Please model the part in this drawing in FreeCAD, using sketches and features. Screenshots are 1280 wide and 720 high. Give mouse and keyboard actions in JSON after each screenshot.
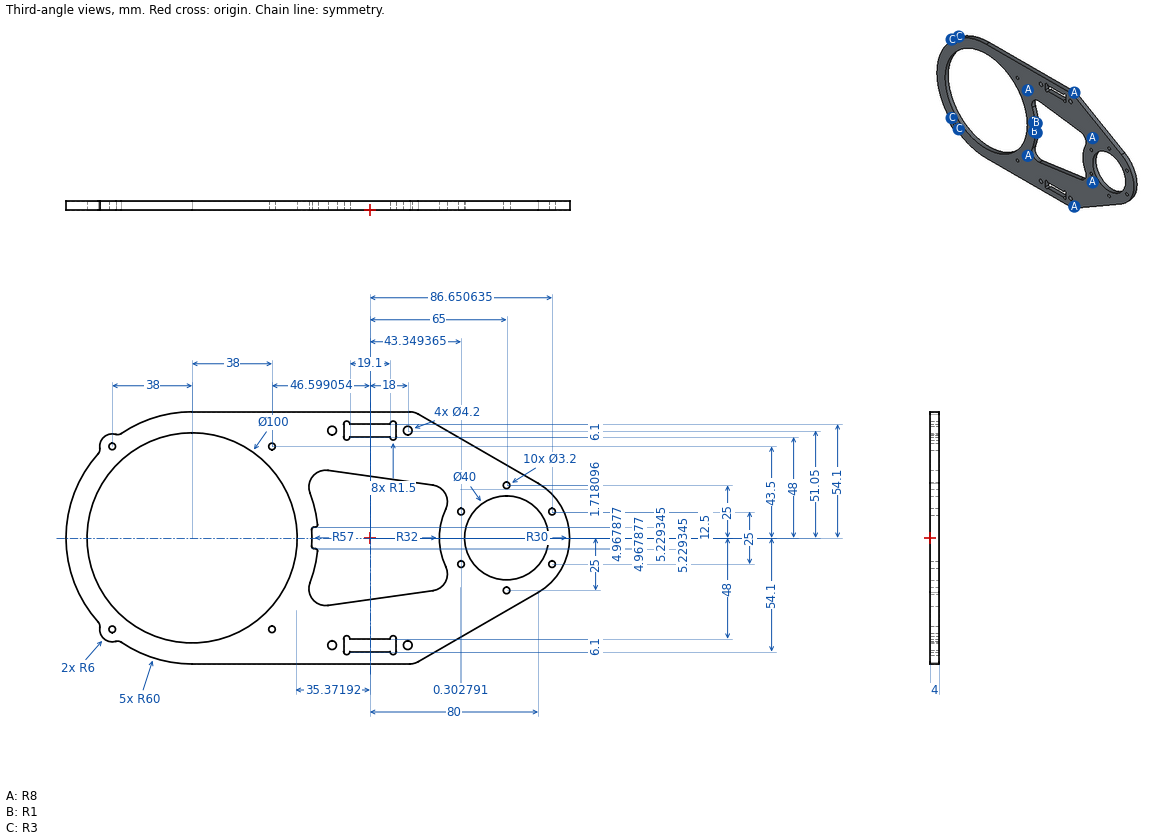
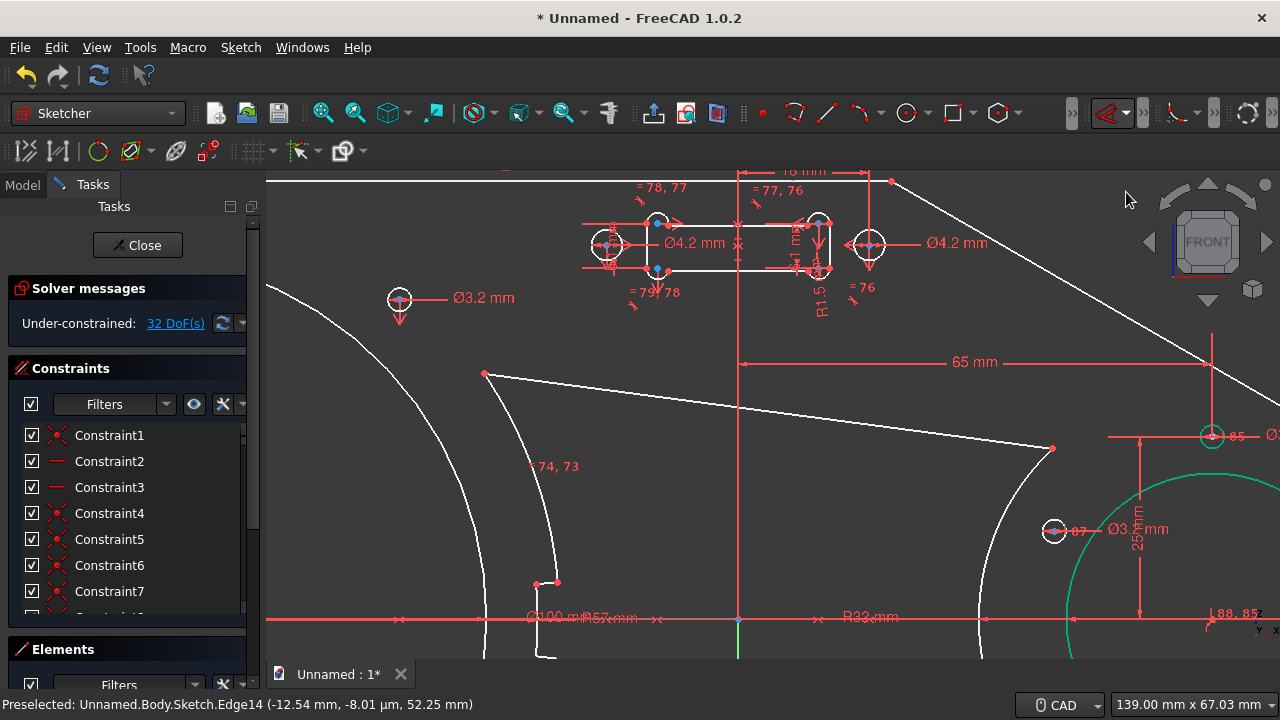
{"action": "scroll", "coordinate": [768, 326], "scroll_direction": "down", "scroll_amount": 6}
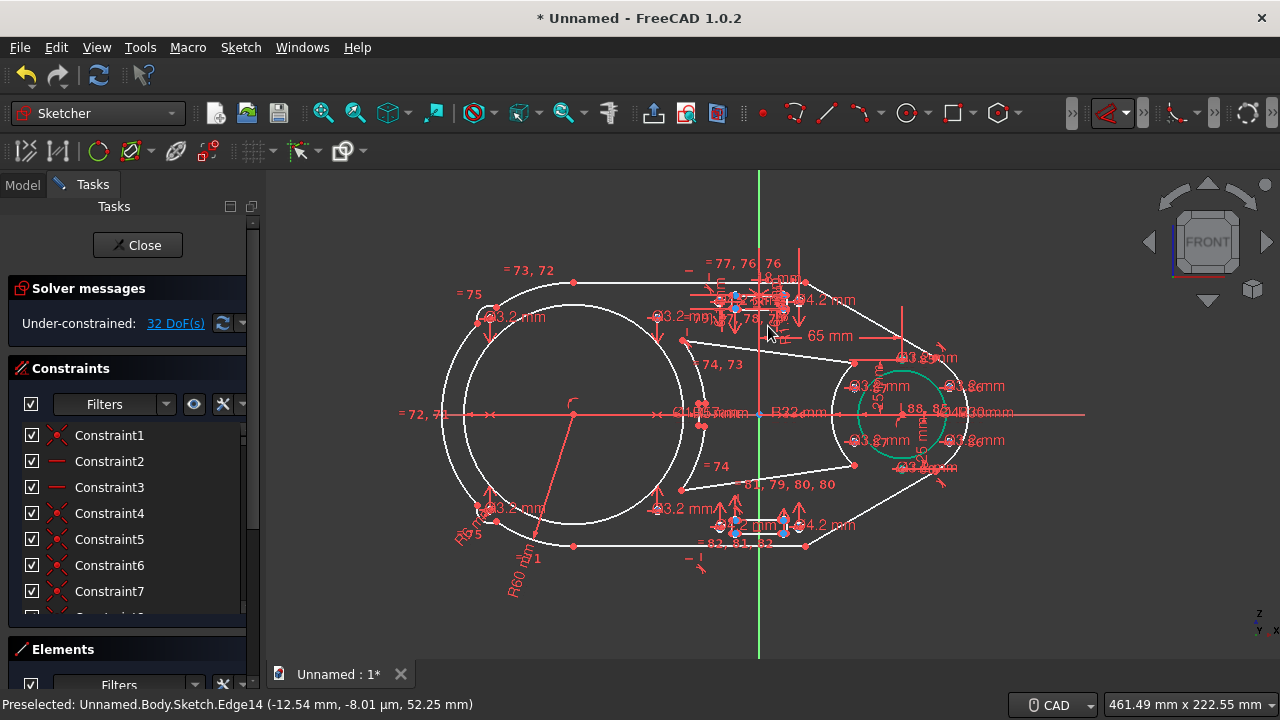
{"action": "scroll", "coordinate": [787, 530], "scroll_direction": "up", "scroll_amount": 7}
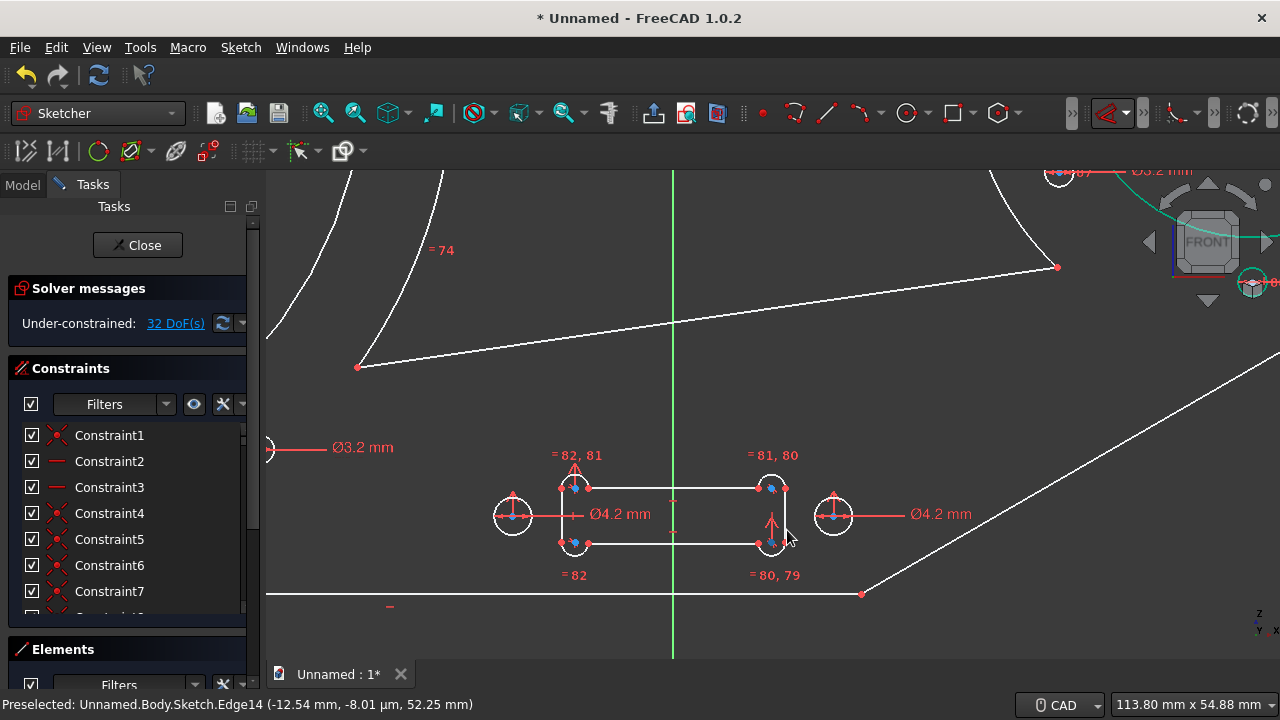
{"action": "left_click", "coordinate": [785, 526]}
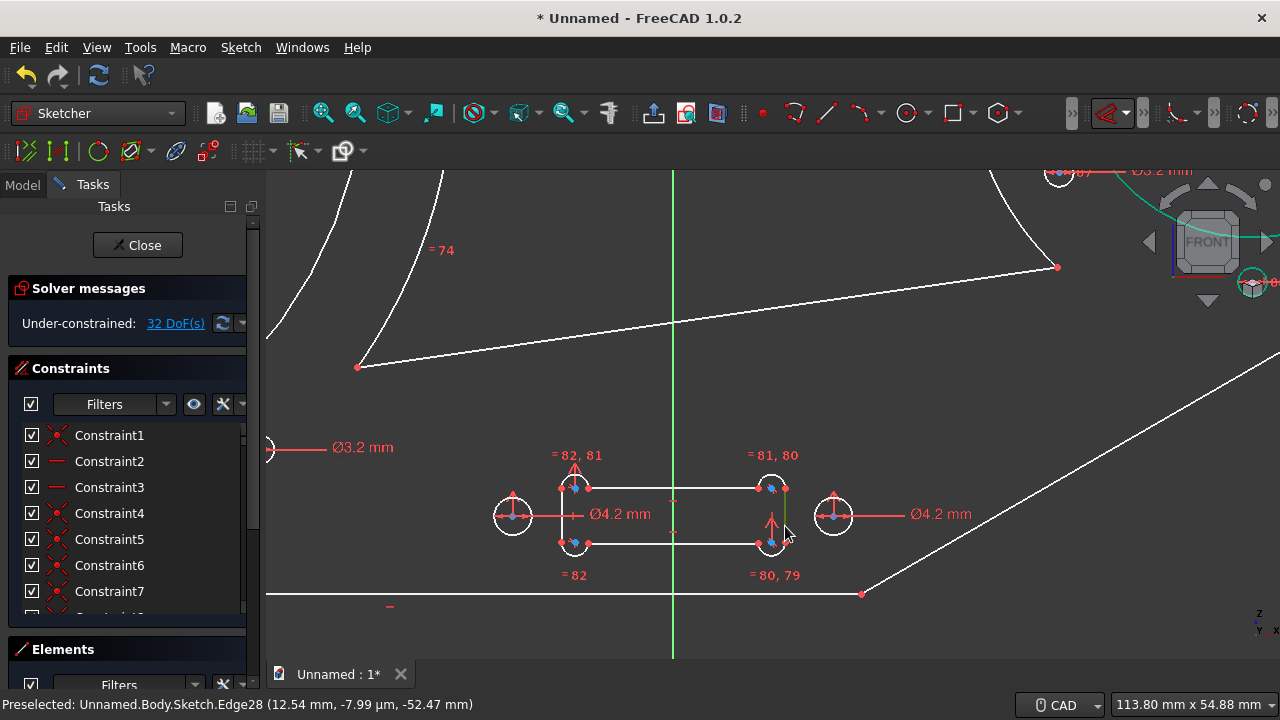
{"action": "key", "text": "i"}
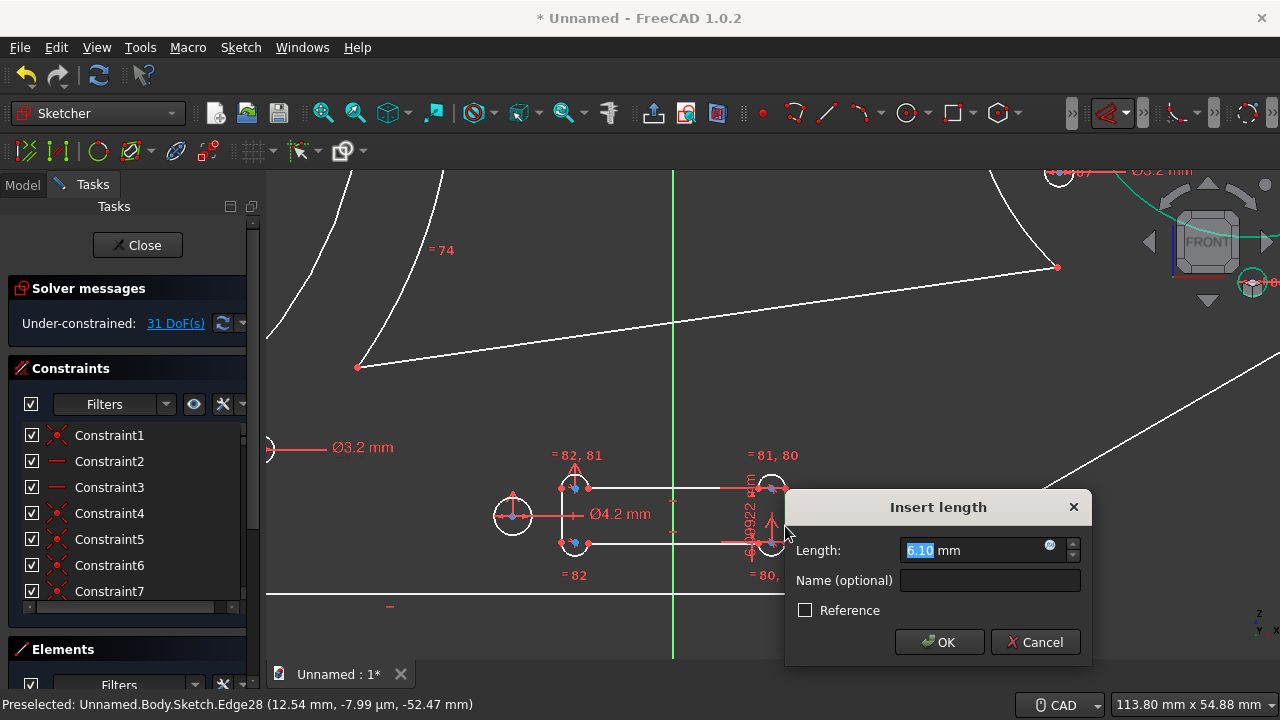
{"action": "type", "text": "6.1"}
{"action": "key", "text": "Return"}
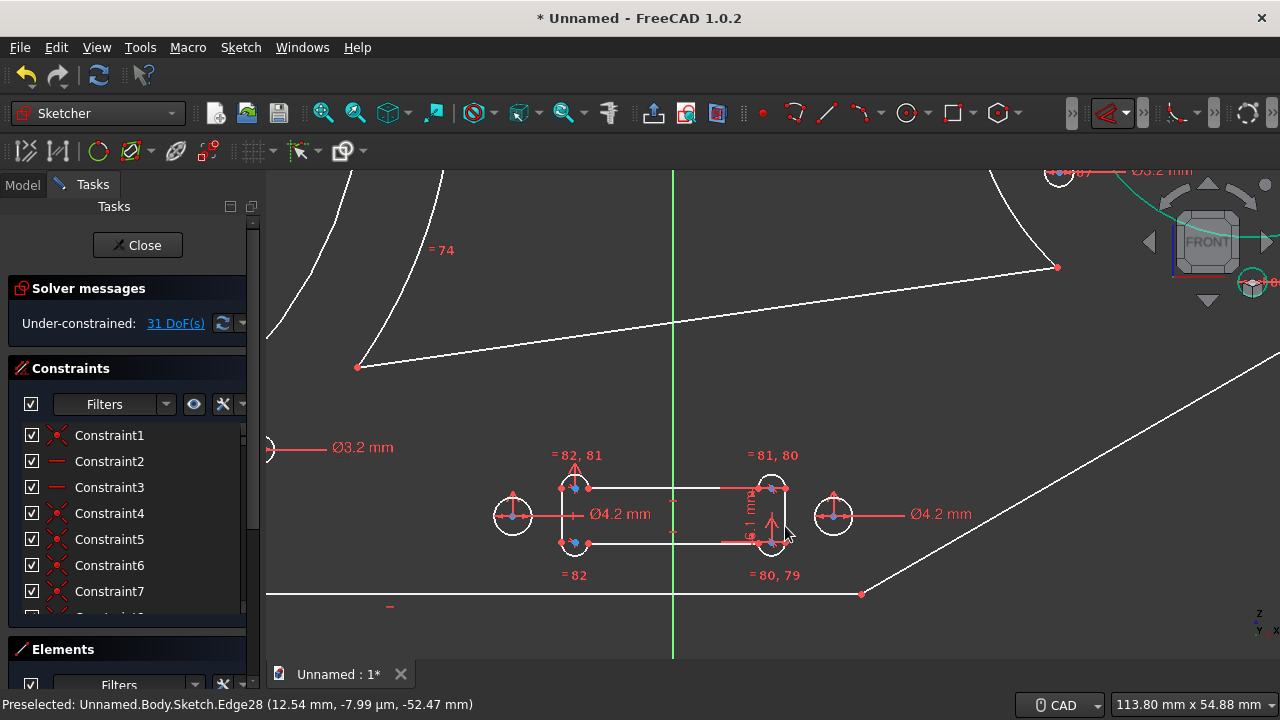
{"action": "left_click", "coordinate": [562, 504]}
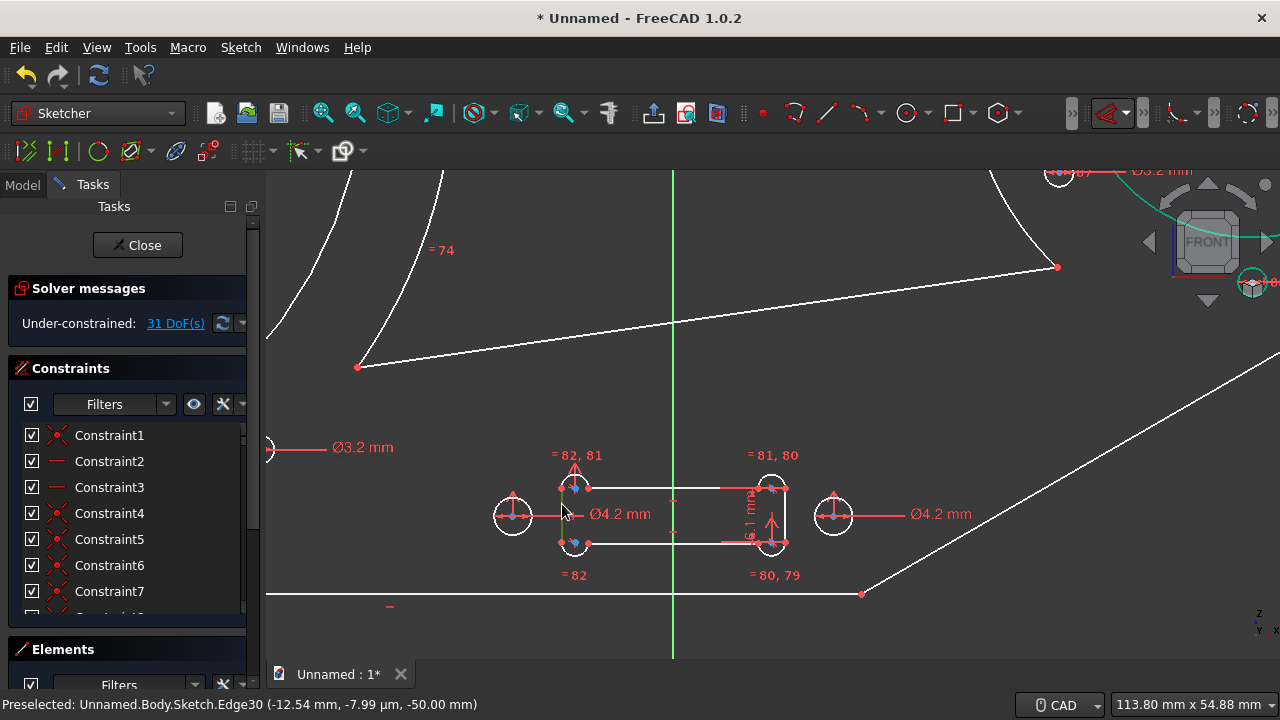
{"action": "left_click", "coordinate": [1128, 114]}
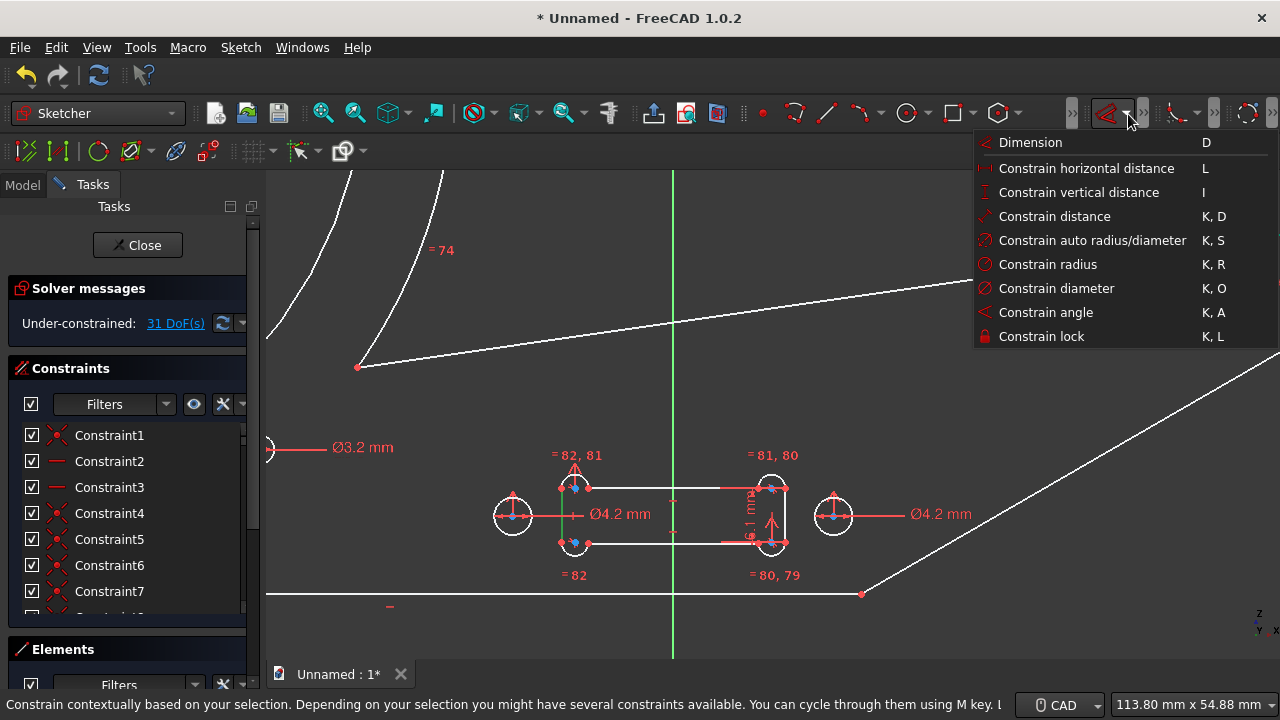
{"action": "left_click", "coordinate": [1126, 192]}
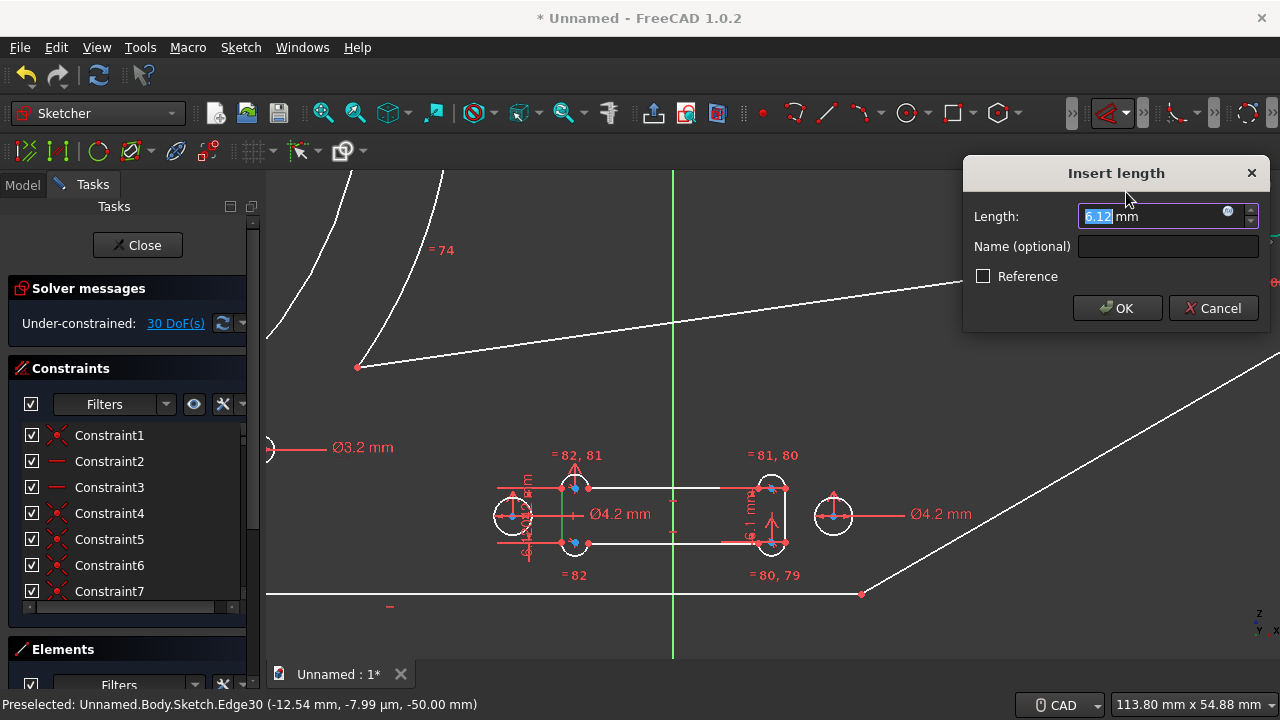
{"action": "type", "text": "6.1"}
{"action": "key", "text": "Return"}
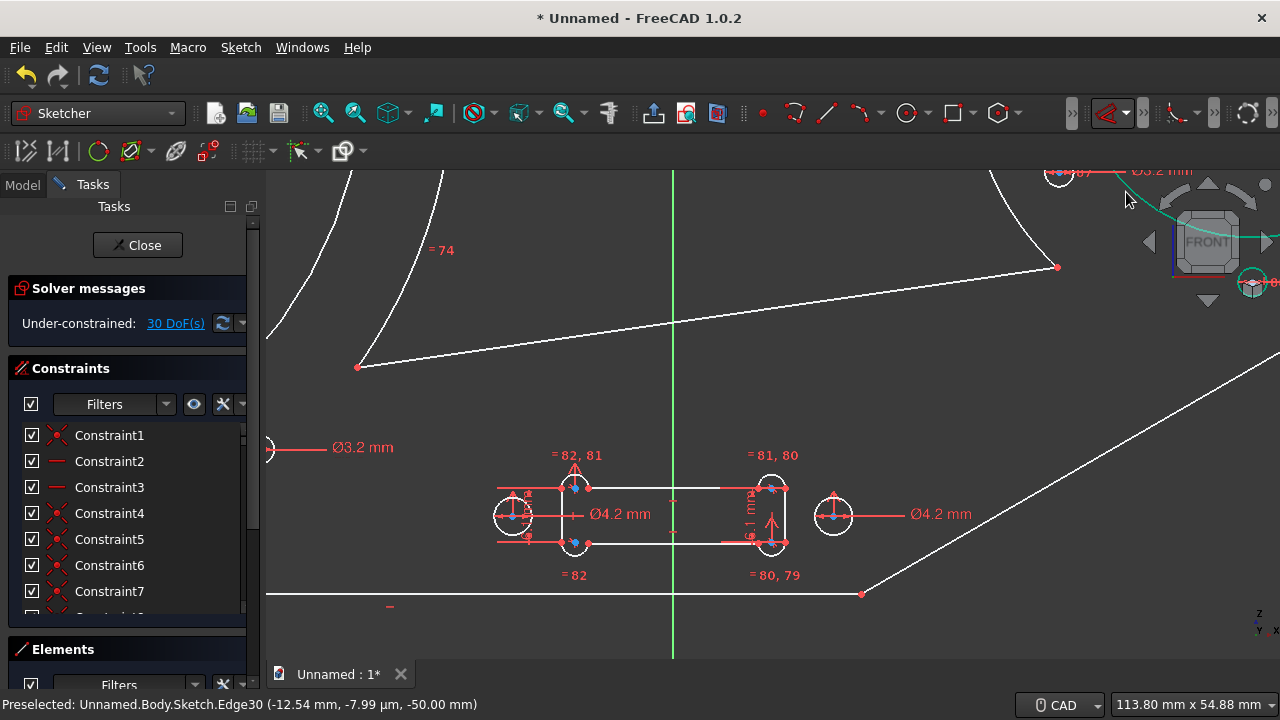
{"action": "scroll", "coordinate": [787, 531], "scroll_direction": "down", "scroll_amount": 7}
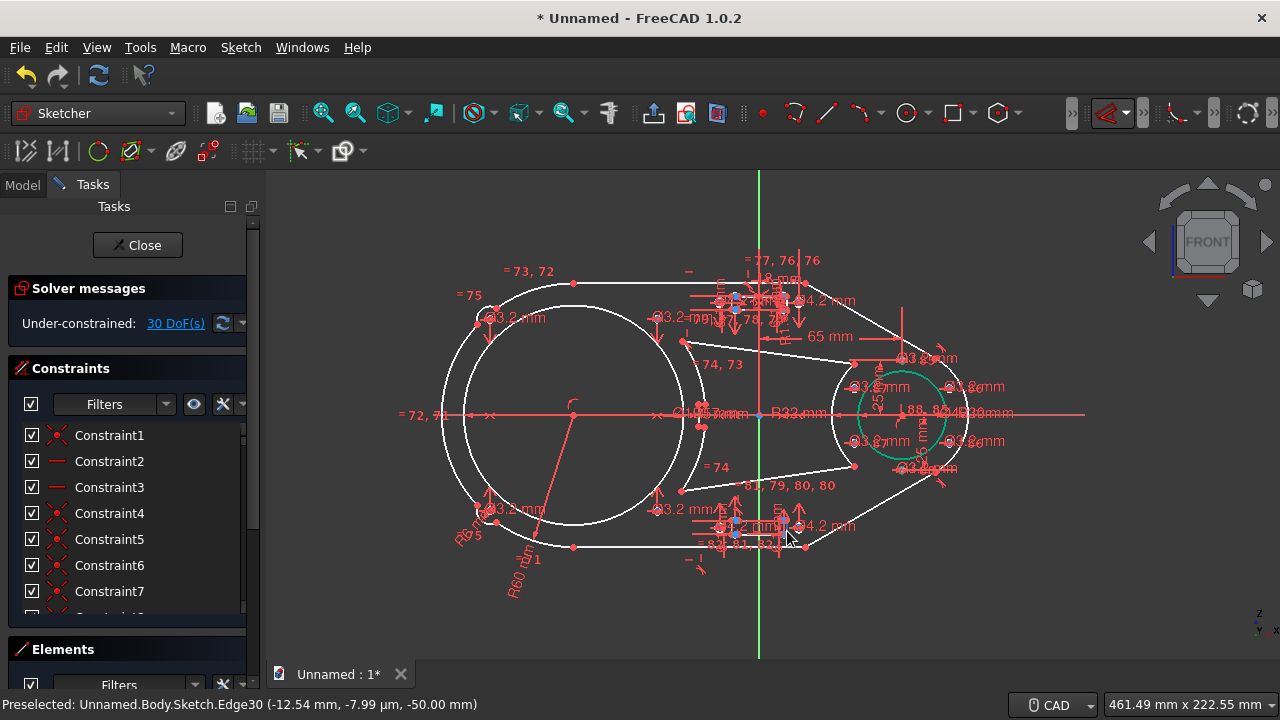
{"action": "left_click", "coordinate": [937, 474]}